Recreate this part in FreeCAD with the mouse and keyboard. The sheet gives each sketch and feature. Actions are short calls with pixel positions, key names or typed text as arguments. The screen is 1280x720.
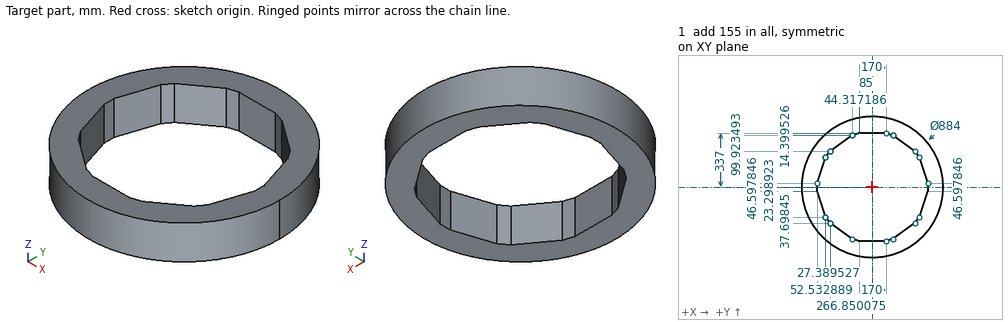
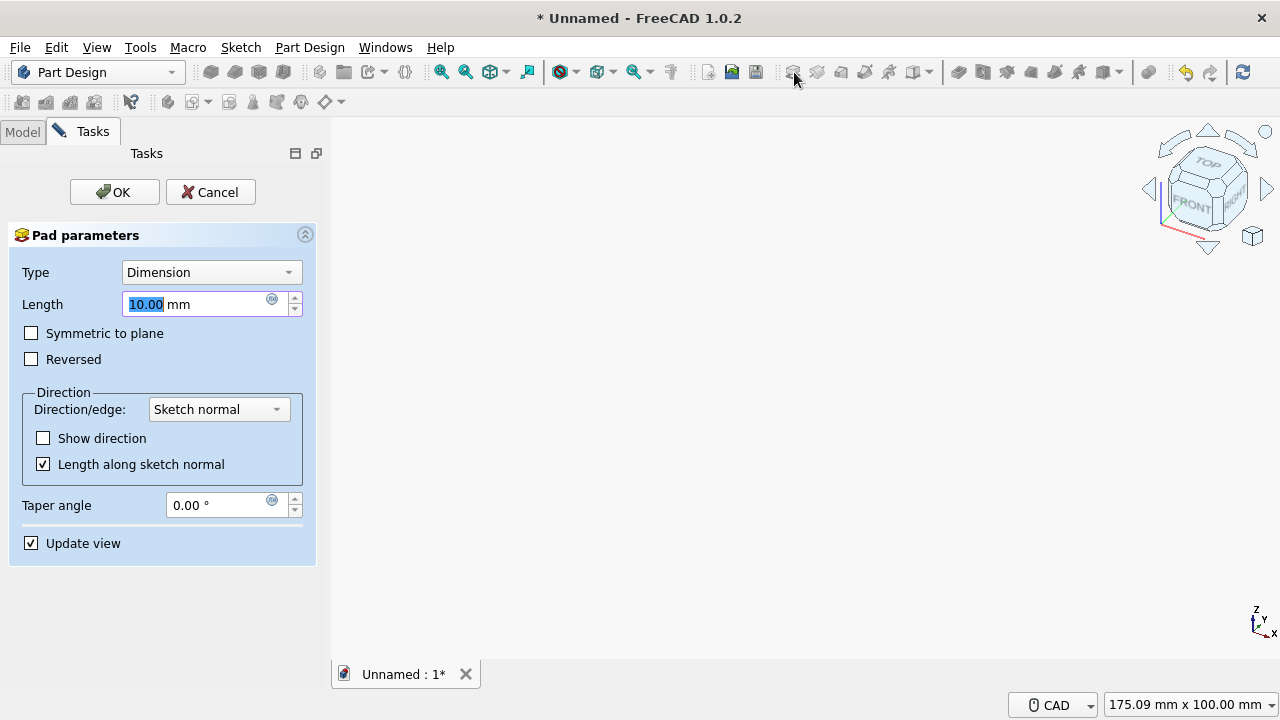
text(155)
key(Tab)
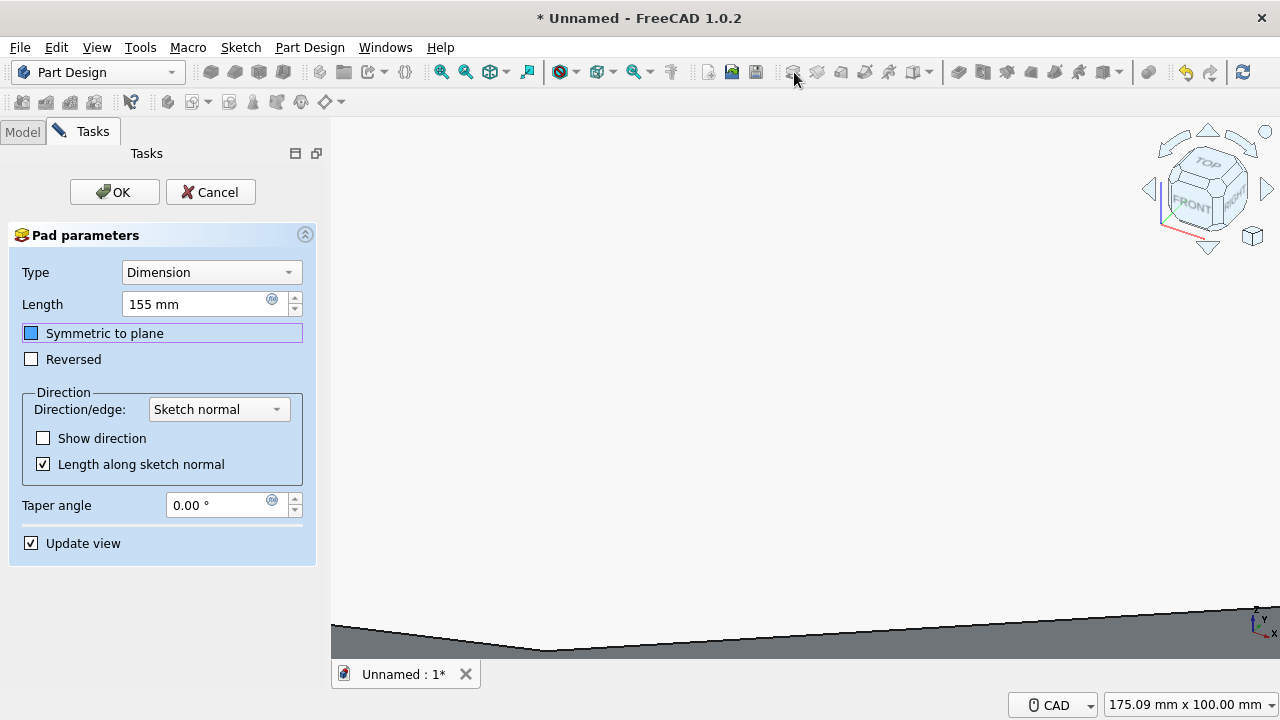
click(30, 333)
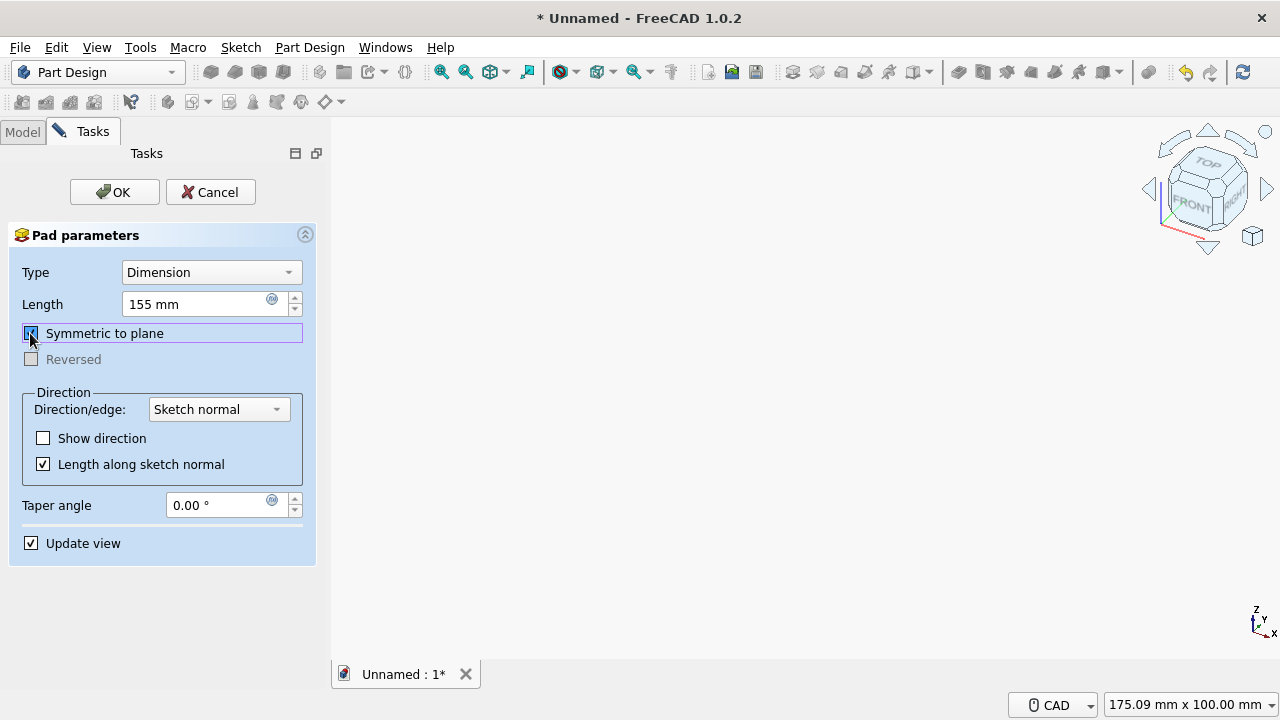
click(115, 192)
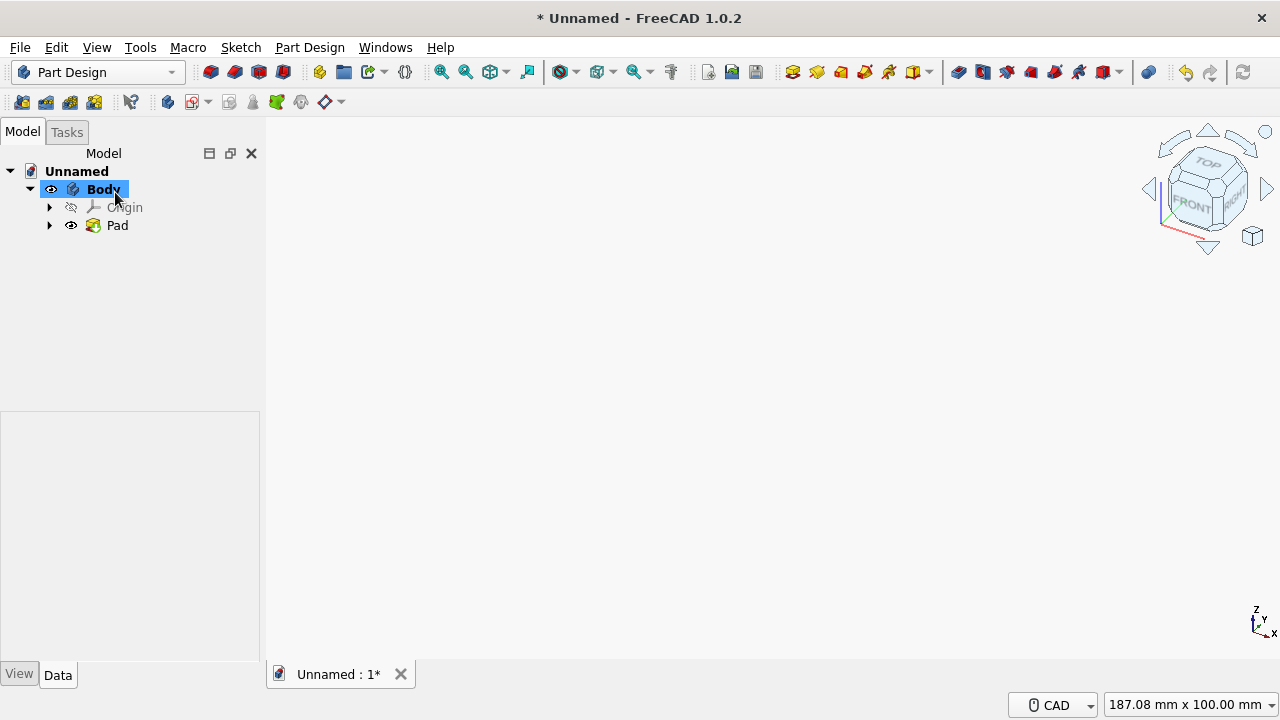
key(0)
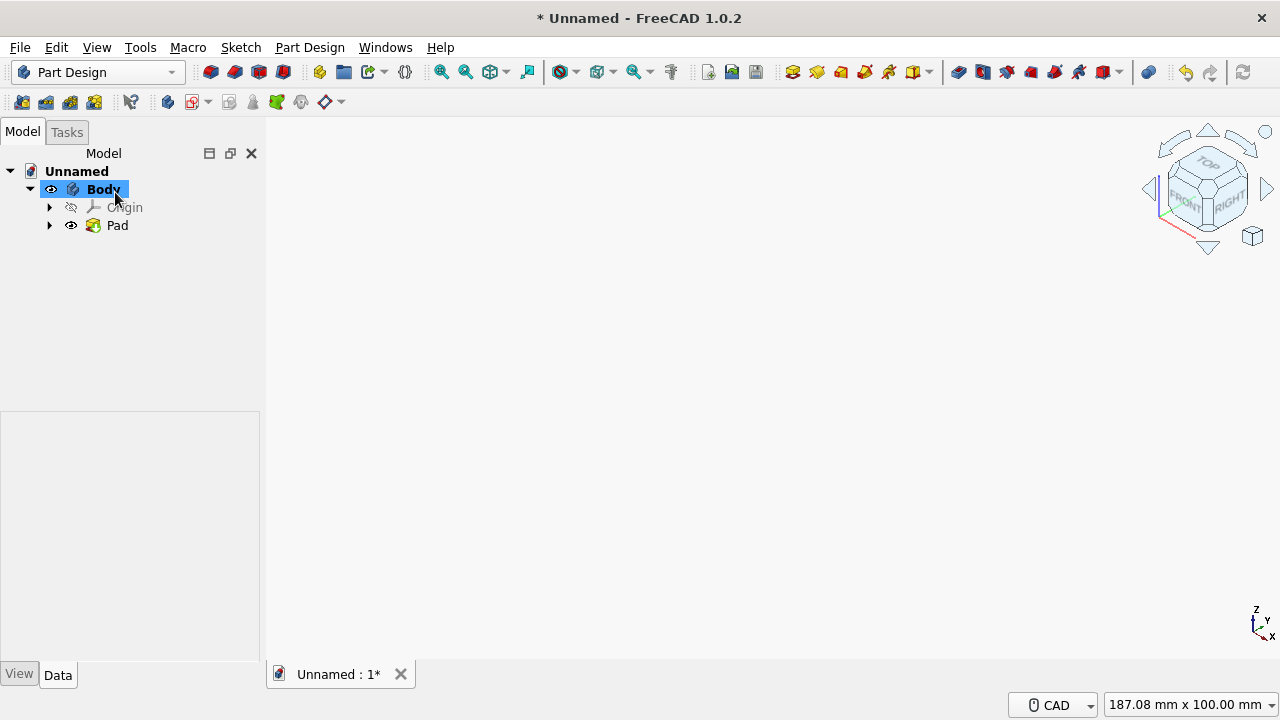
click(442, 72)